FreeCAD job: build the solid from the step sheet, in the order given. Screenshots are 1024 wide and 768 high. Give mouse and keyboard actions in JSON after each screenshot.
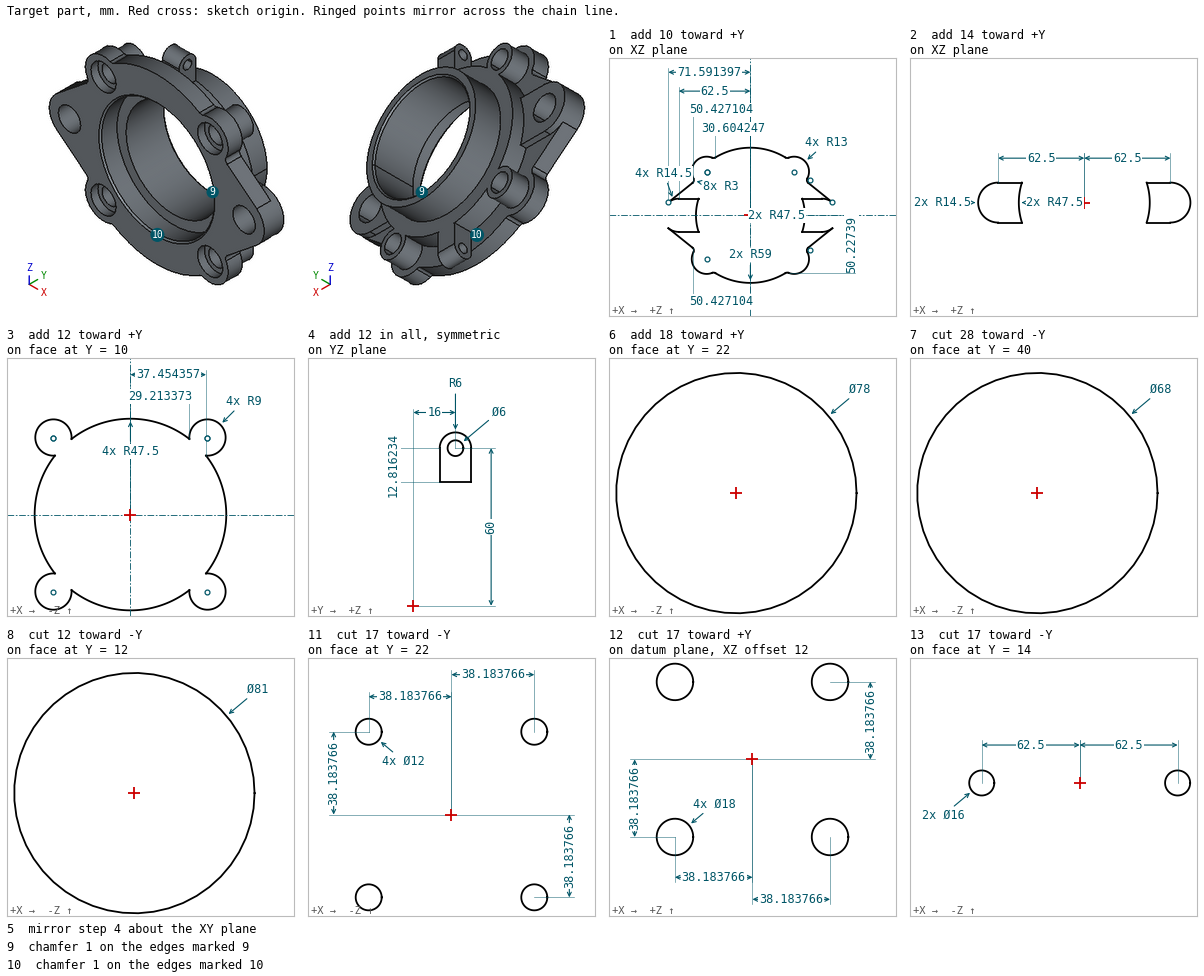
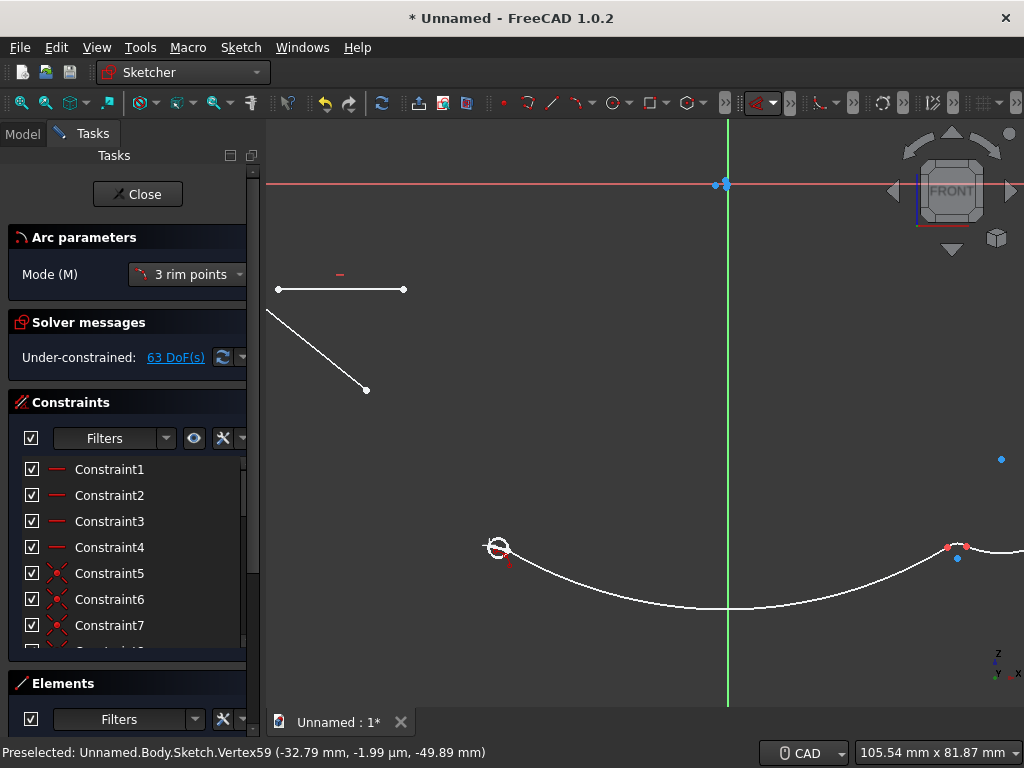
{"action": "scroll", "coordinate": [499, 543], "scroll_direction": "up", "scroll_amount": 10}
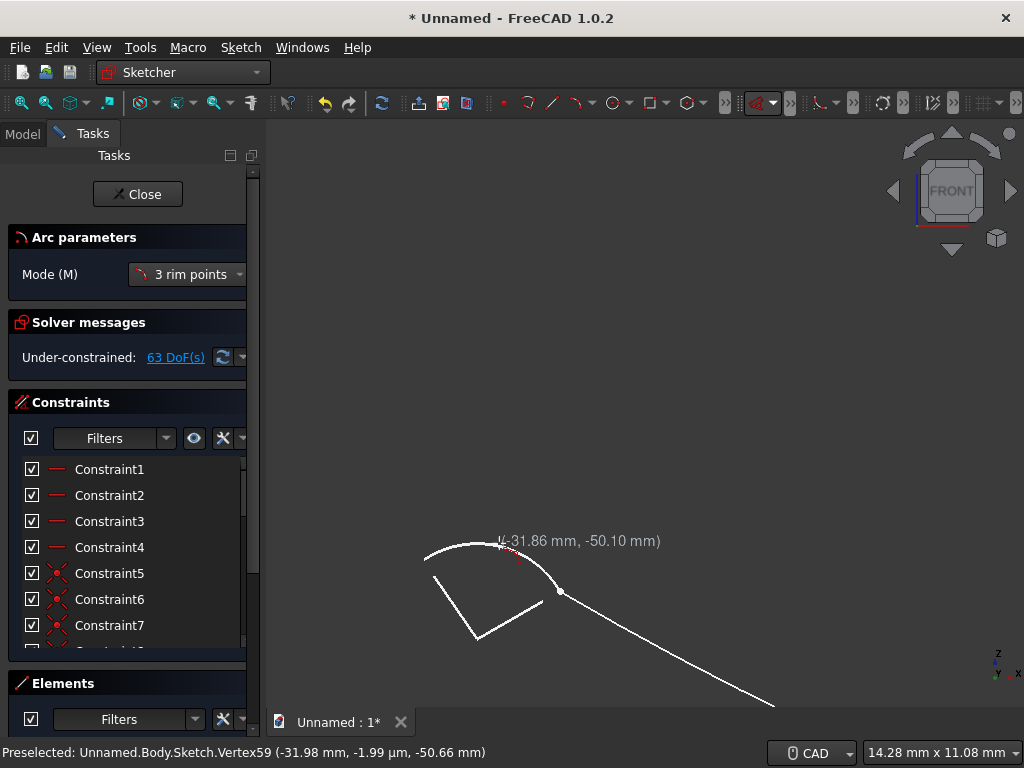
{"action": "left_click", "coordinate": [494, 541]}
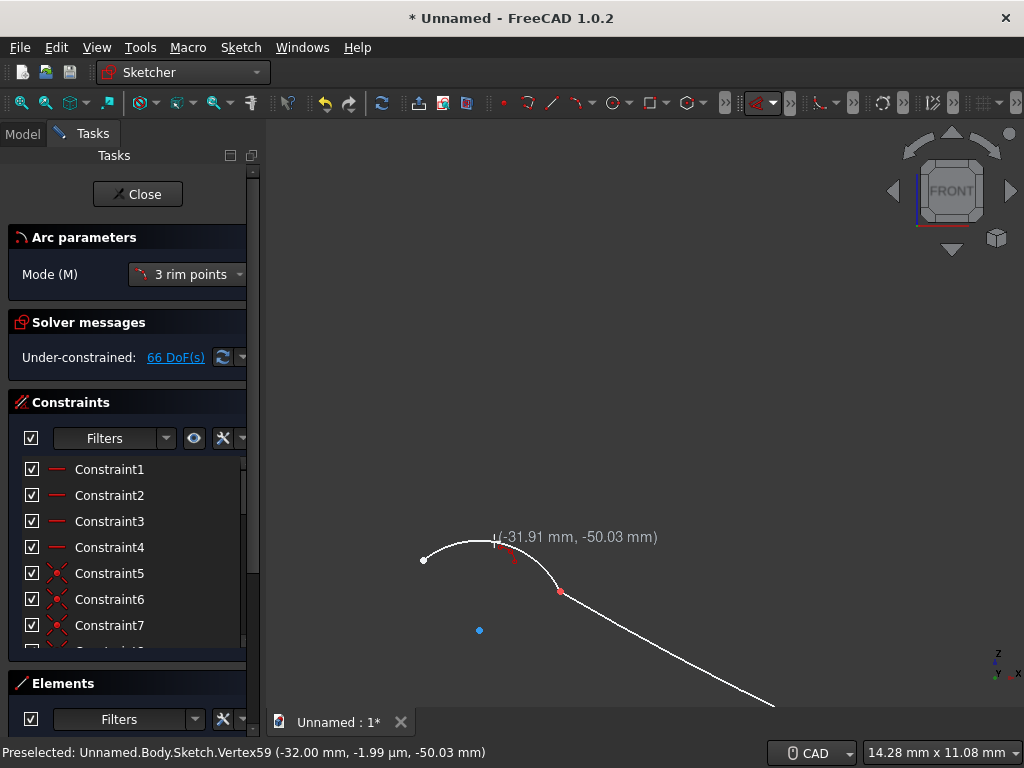
{"action": "scroll", "coordinate": [492, 545], "scroll_direction": "down", "scroll_amount": 15}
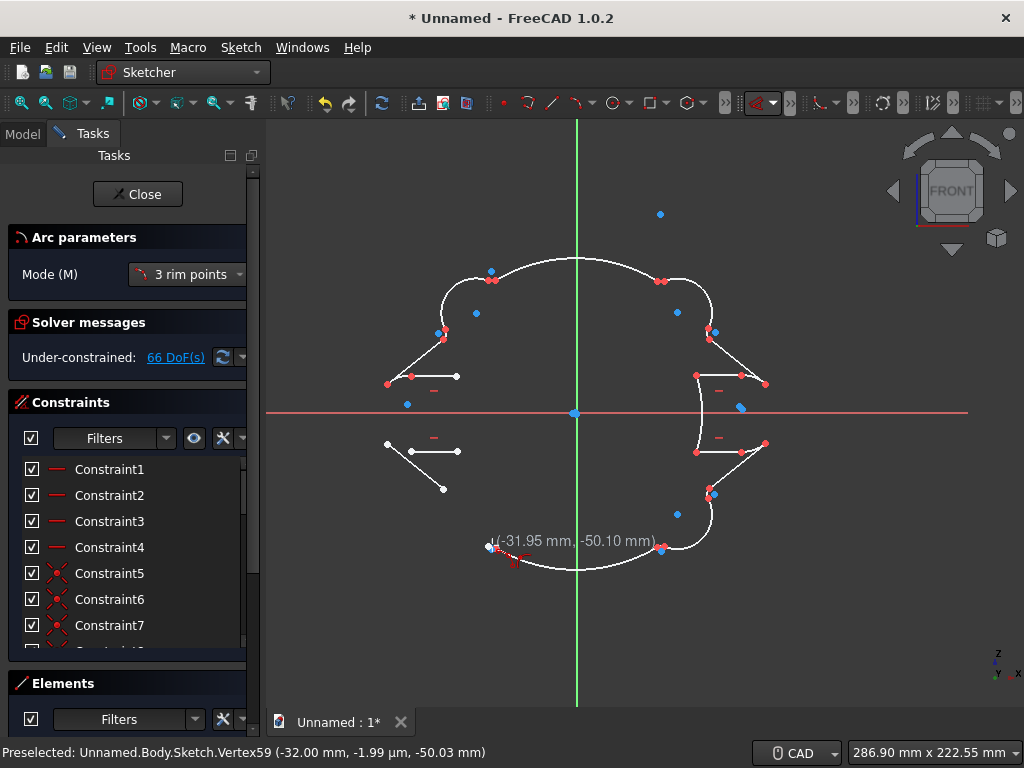
{"action": "scroll", "coordinate": [489, 546], "scroll_direction": "up", "scroll_amount": 5}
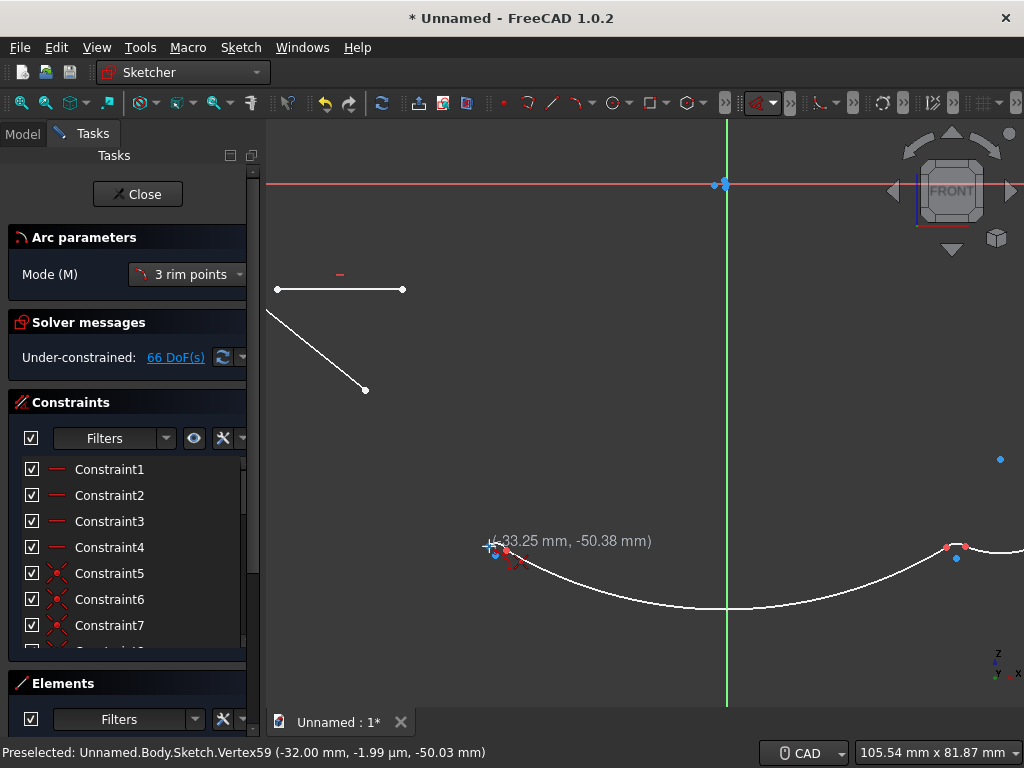
{"action": "left_click", "coordinate": [488, 546]}
{"action": "left_click", "coordinate": [370, 415]}
{"action": "left_click", "coordinate": [383, 521]}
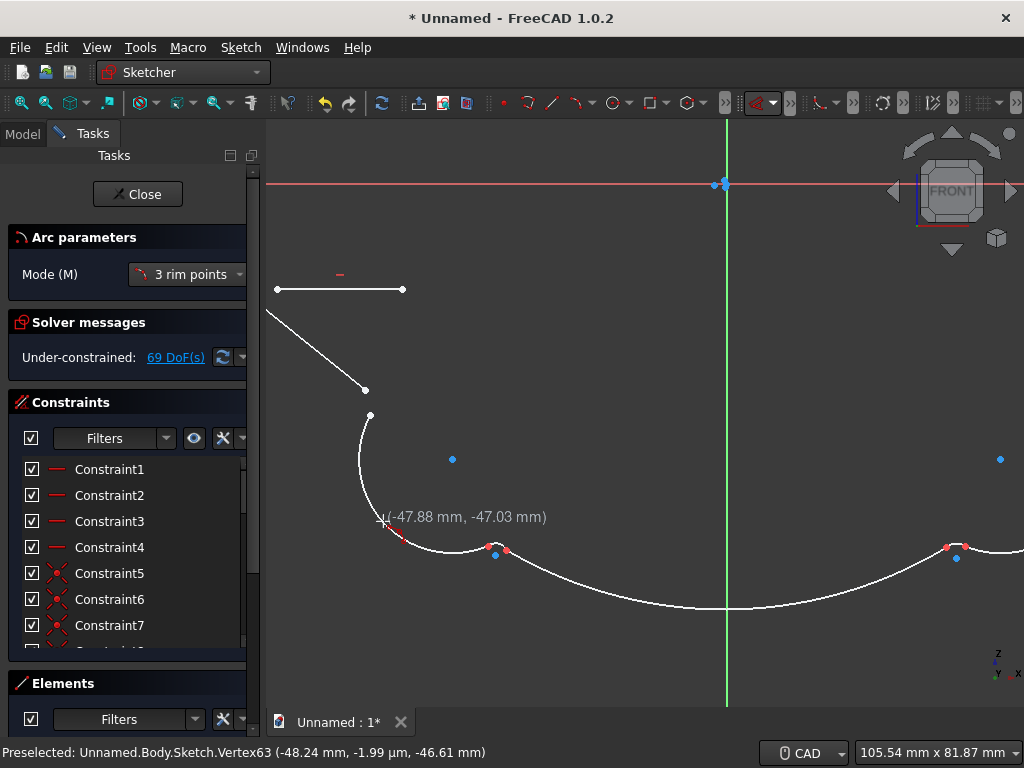
{"action": "left_click", "coordinate": [370, 416]}
{"action": "left_click", "coordinate": [366, 390]}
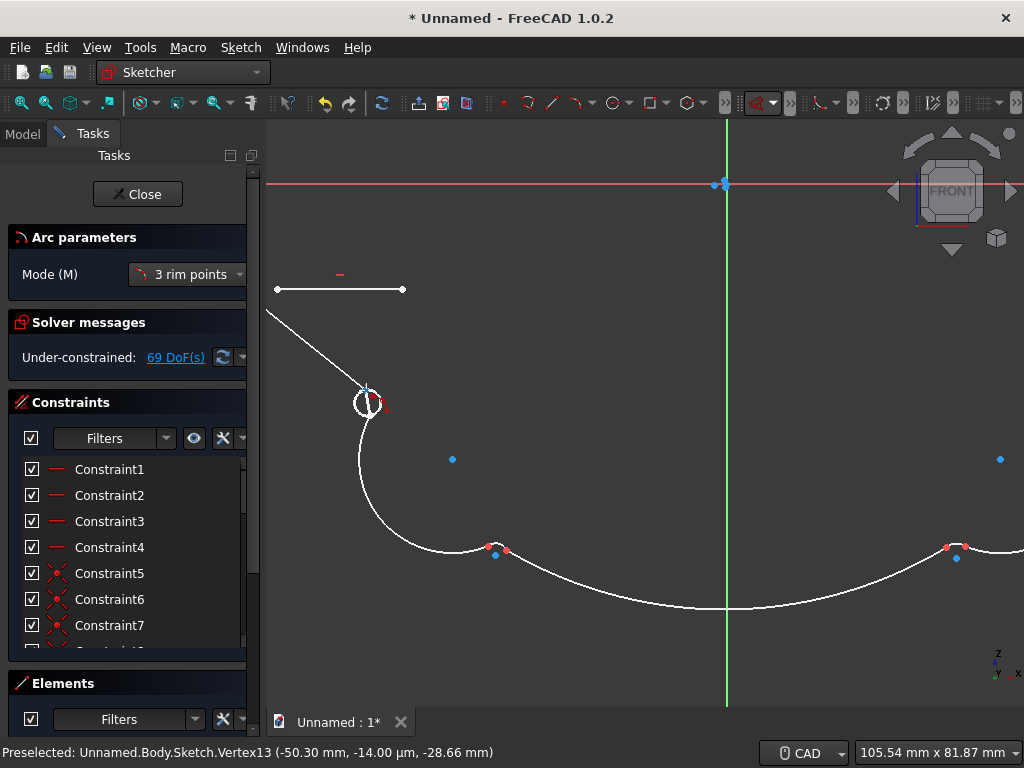
{"action": "scroll", "coordinate": [372, 400], "scroll_direction": "up", "scroll_amount": 6}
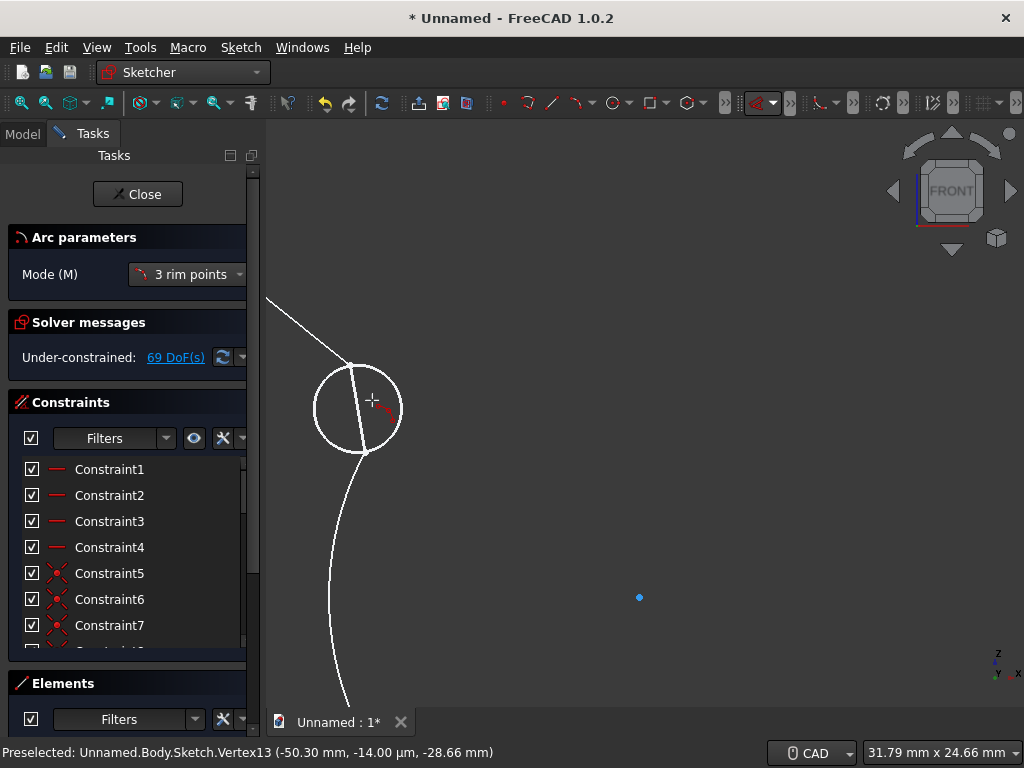
{"action": "left_click", "coordinate": [373, 399]}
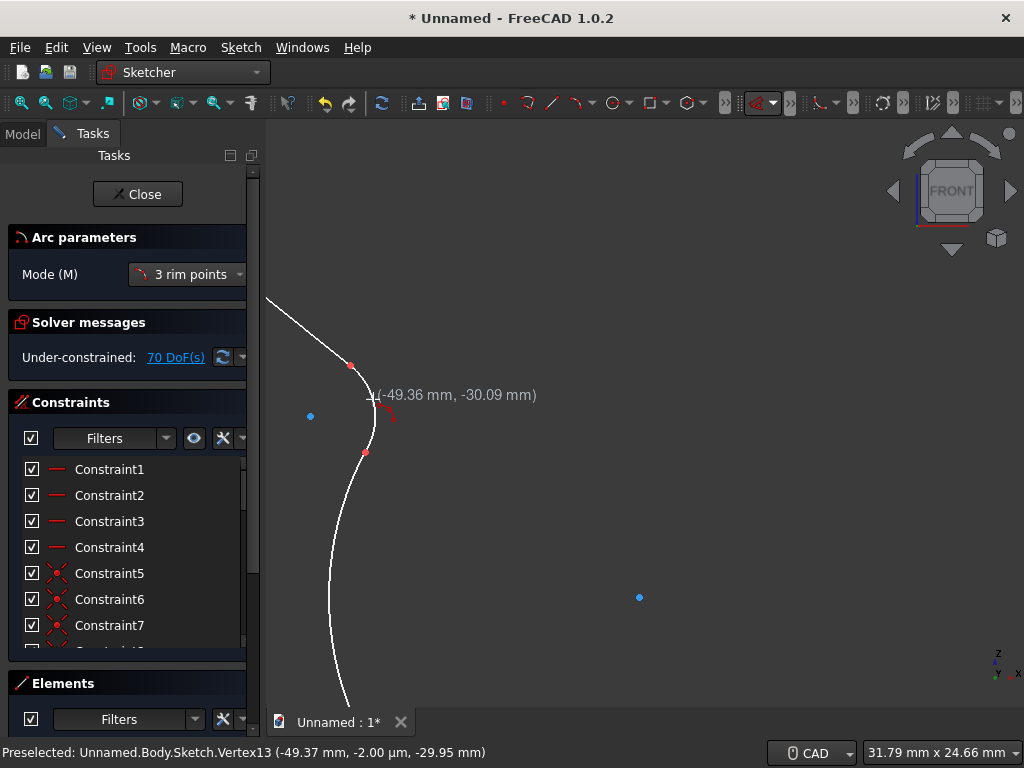
{"action": "scroll", "coordinate": [455, 504], "scroll_direction": "down", "scroll_amount": 11}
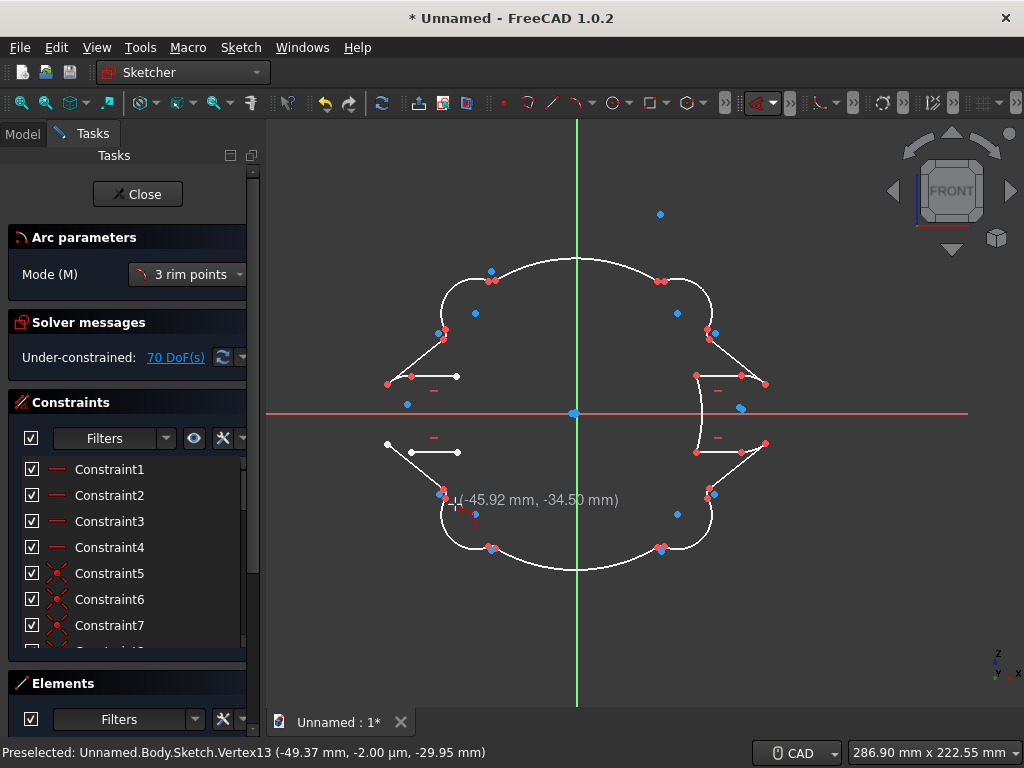
{"action": "left_click", "coordinate": [388, 444]}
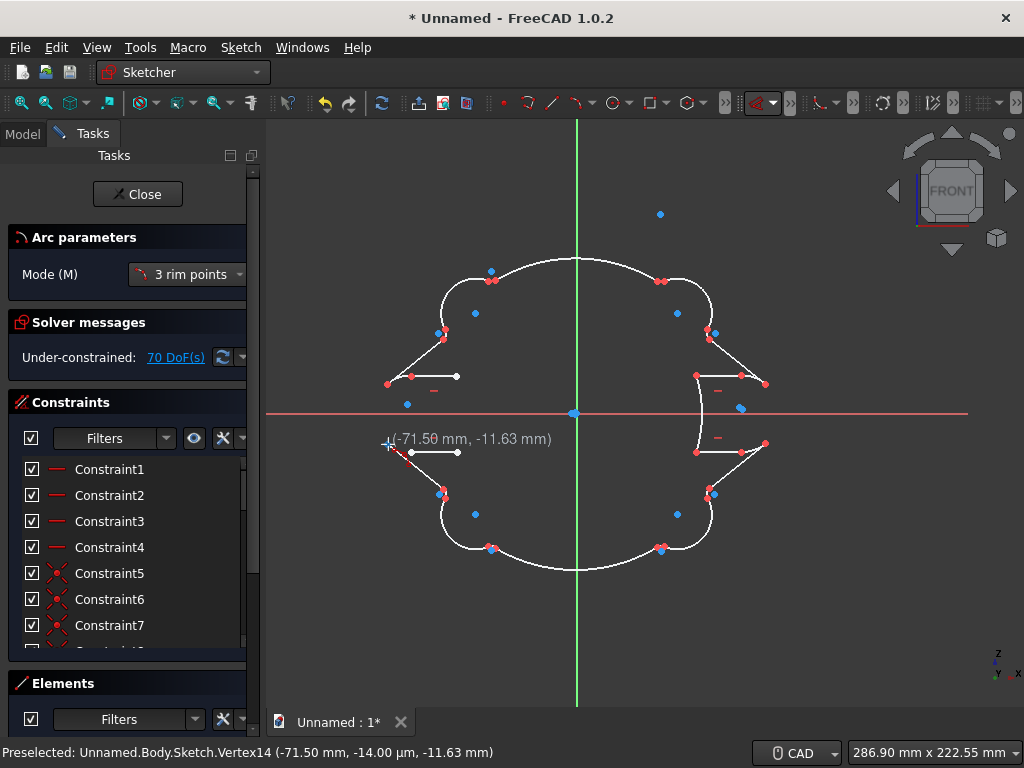
{"action": "scroll", "coordinate": [411, 452], "scroll_direction": "up", "scroll_amount": 4}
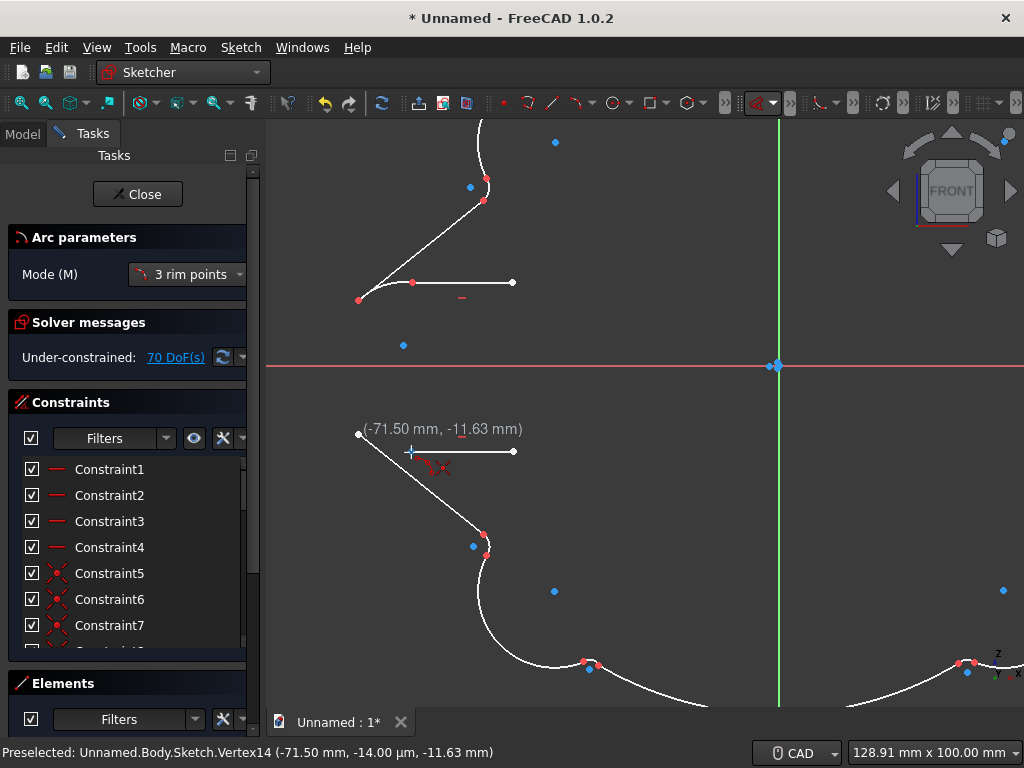
{"action": "left_click", "coordinate": [411, 452]}